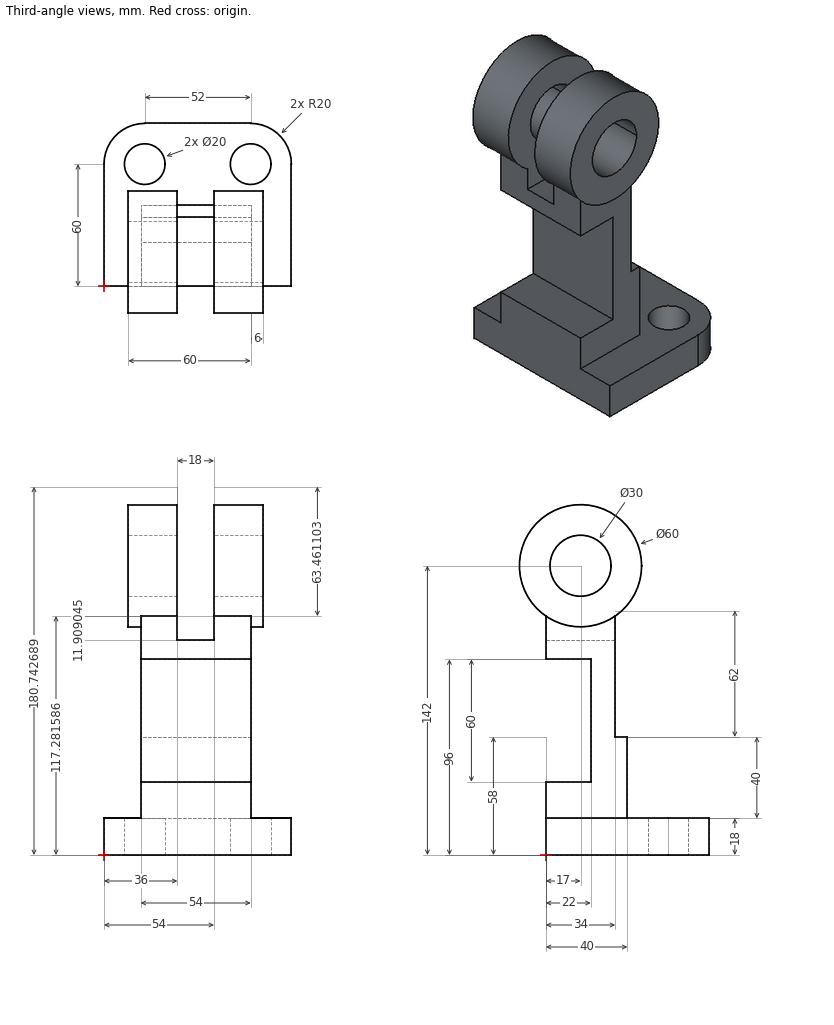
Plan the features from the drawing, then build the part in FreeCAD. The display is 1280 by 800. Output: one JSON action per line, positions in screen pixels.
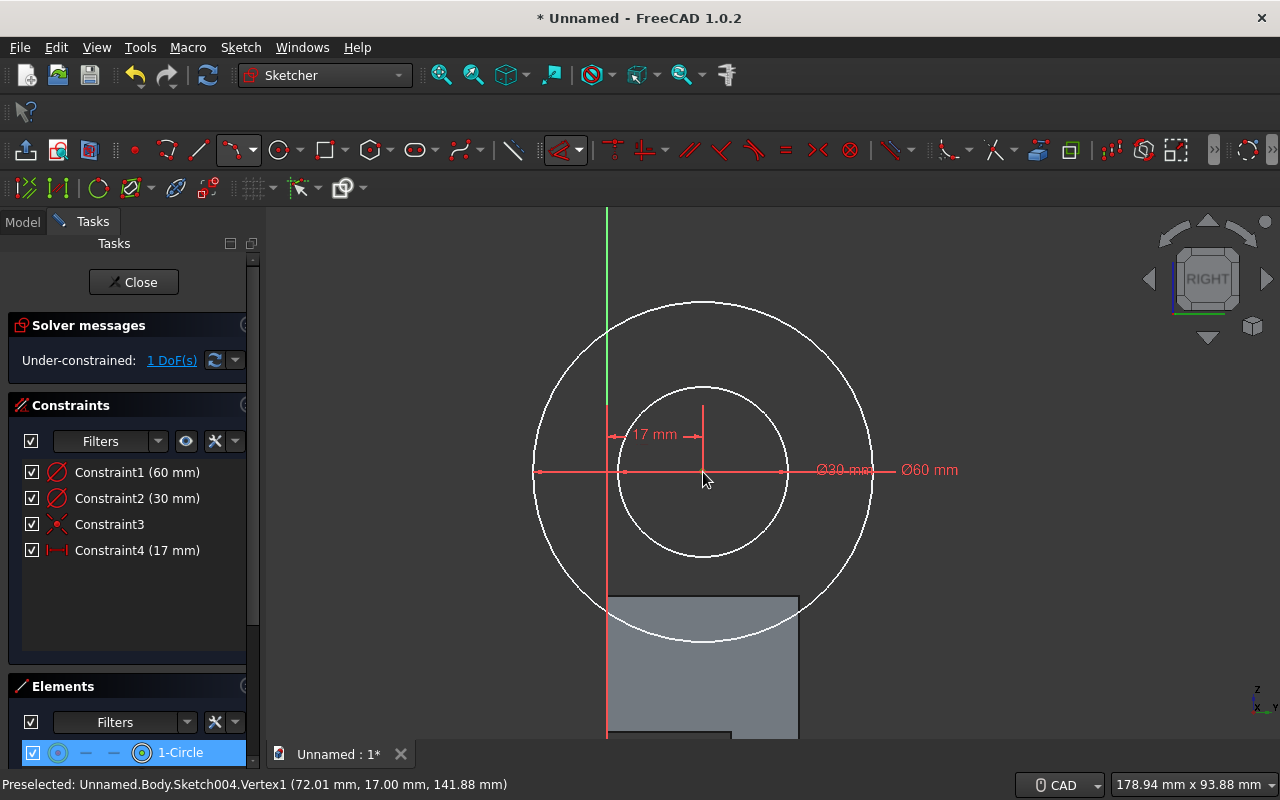
{"action": "left_click", "coordinate": [582, 150]}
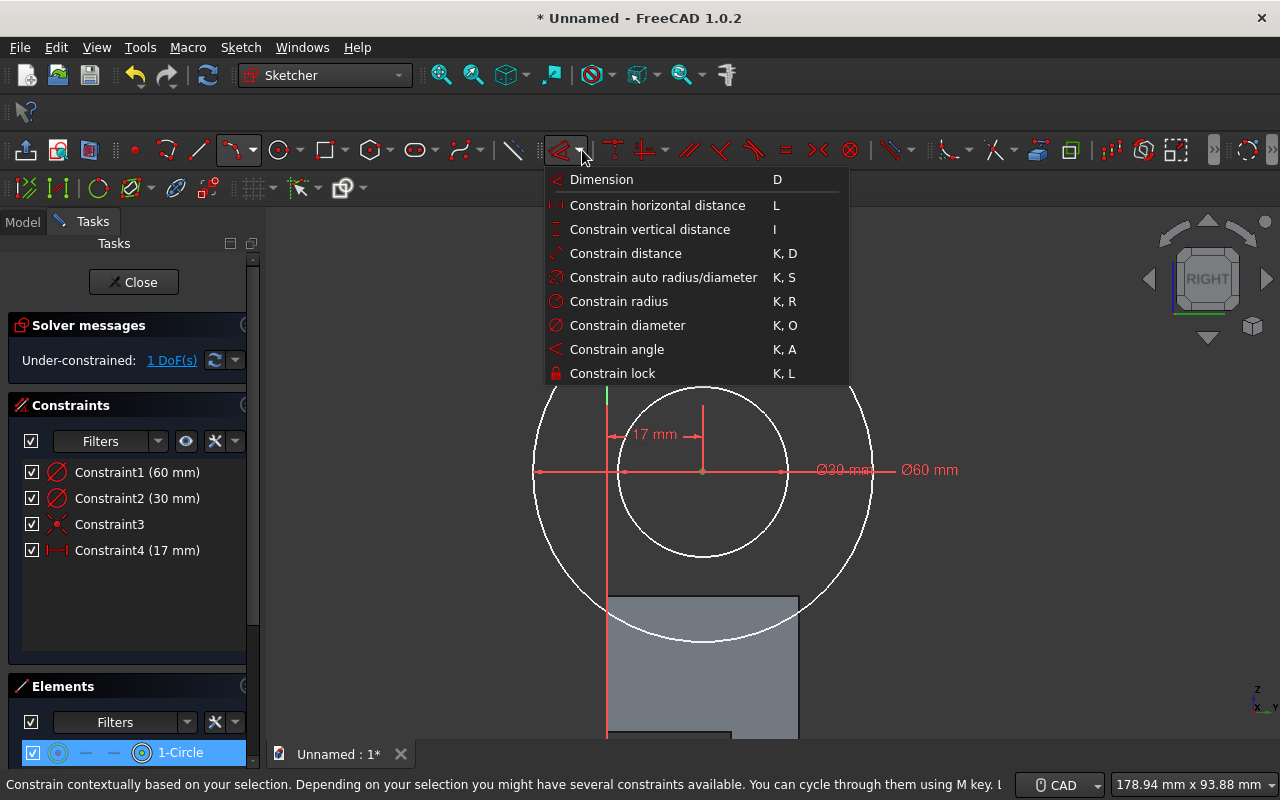
{"action": "left_click", "coordinate": [697, 229]}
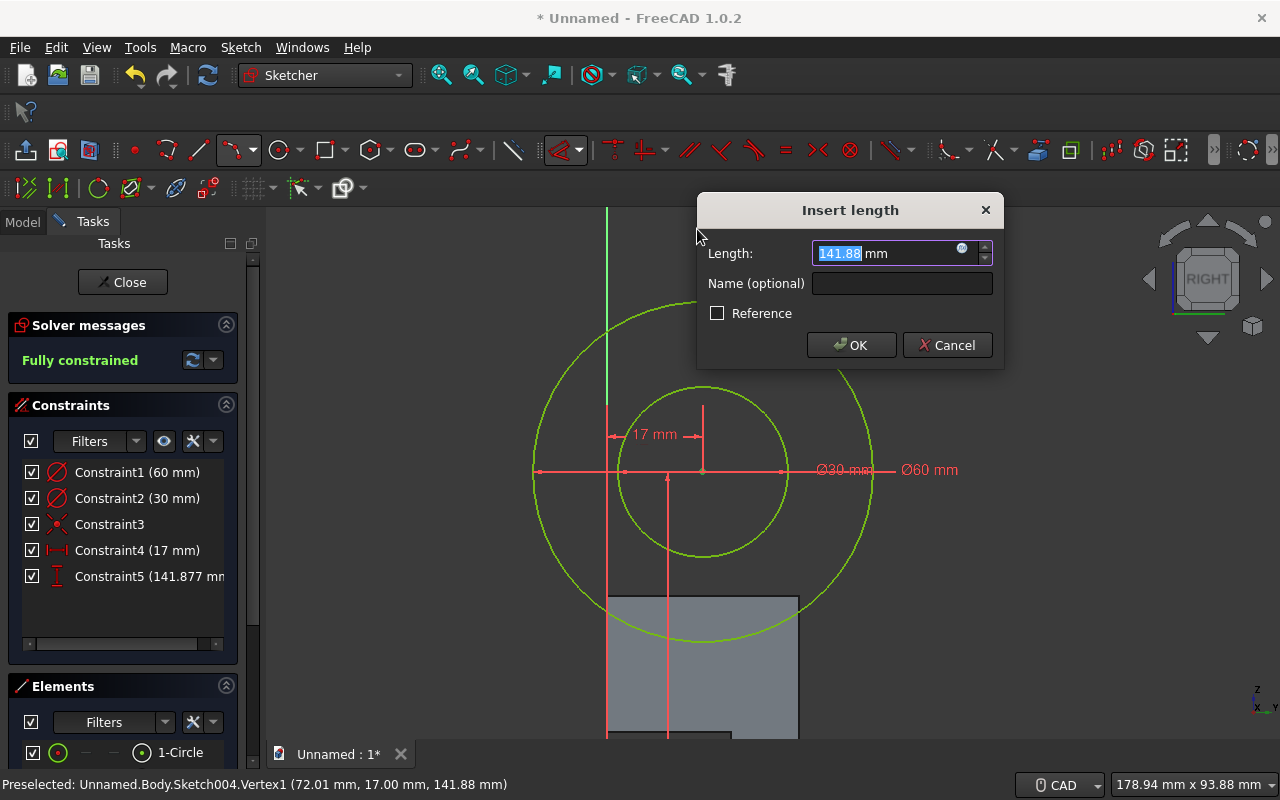
{"action": "type", "text": "142"}
{"action": "key", "text": "Return"}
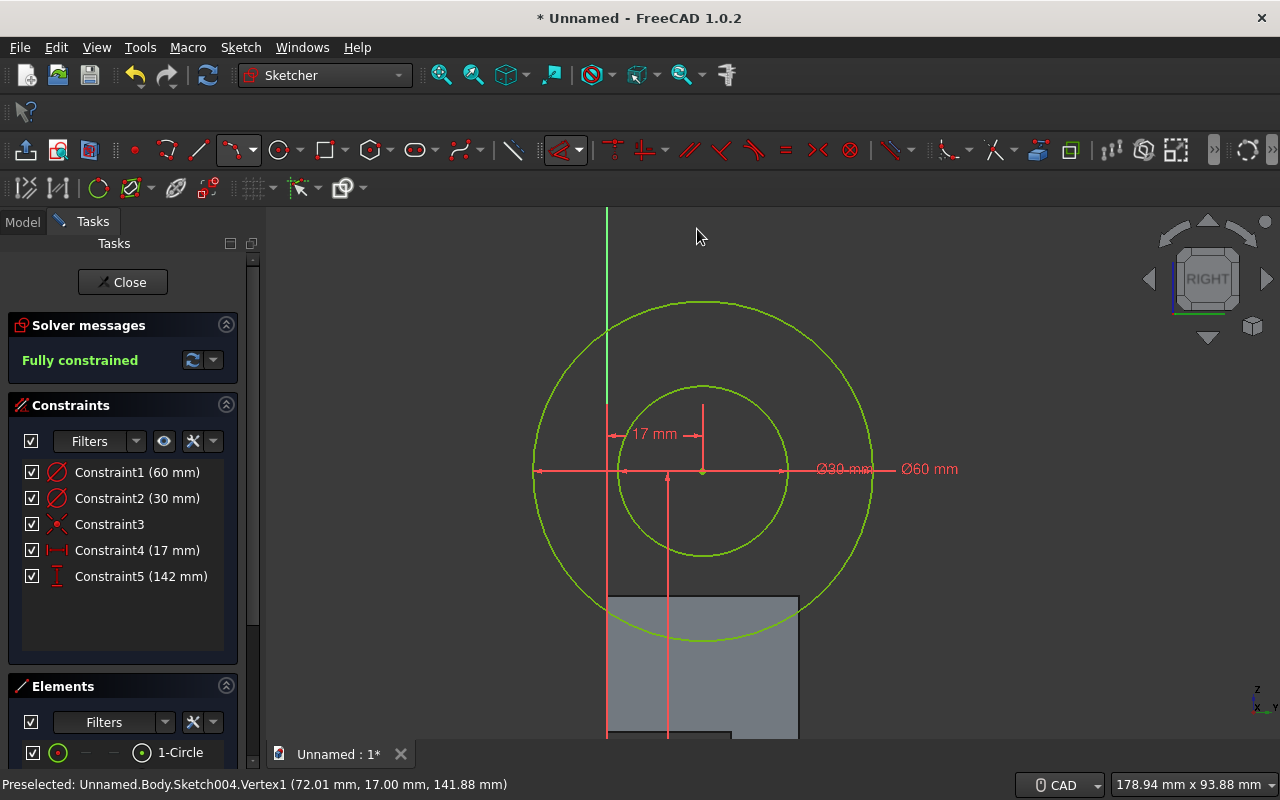
{"action": "left_click", "coordinate": [123, 282]}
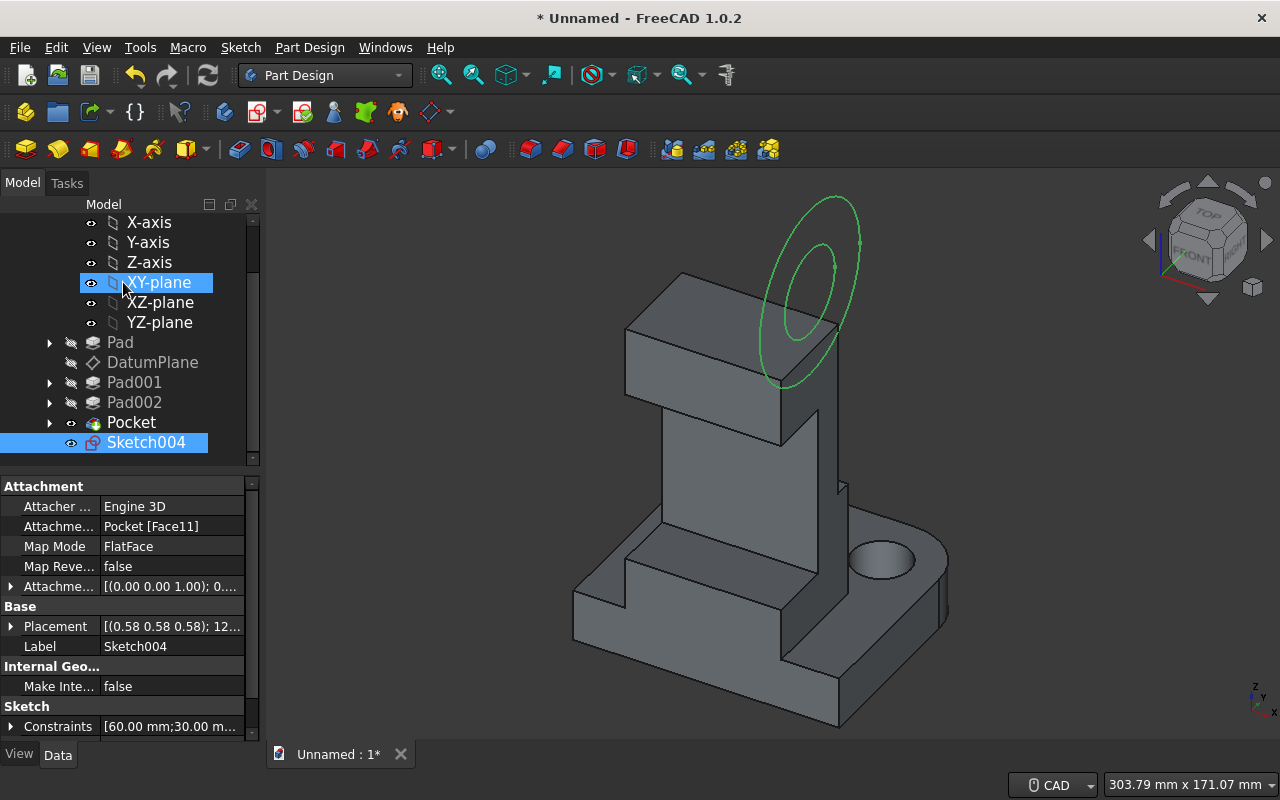
{"action": "left_click", "coordinate": [26, 150]}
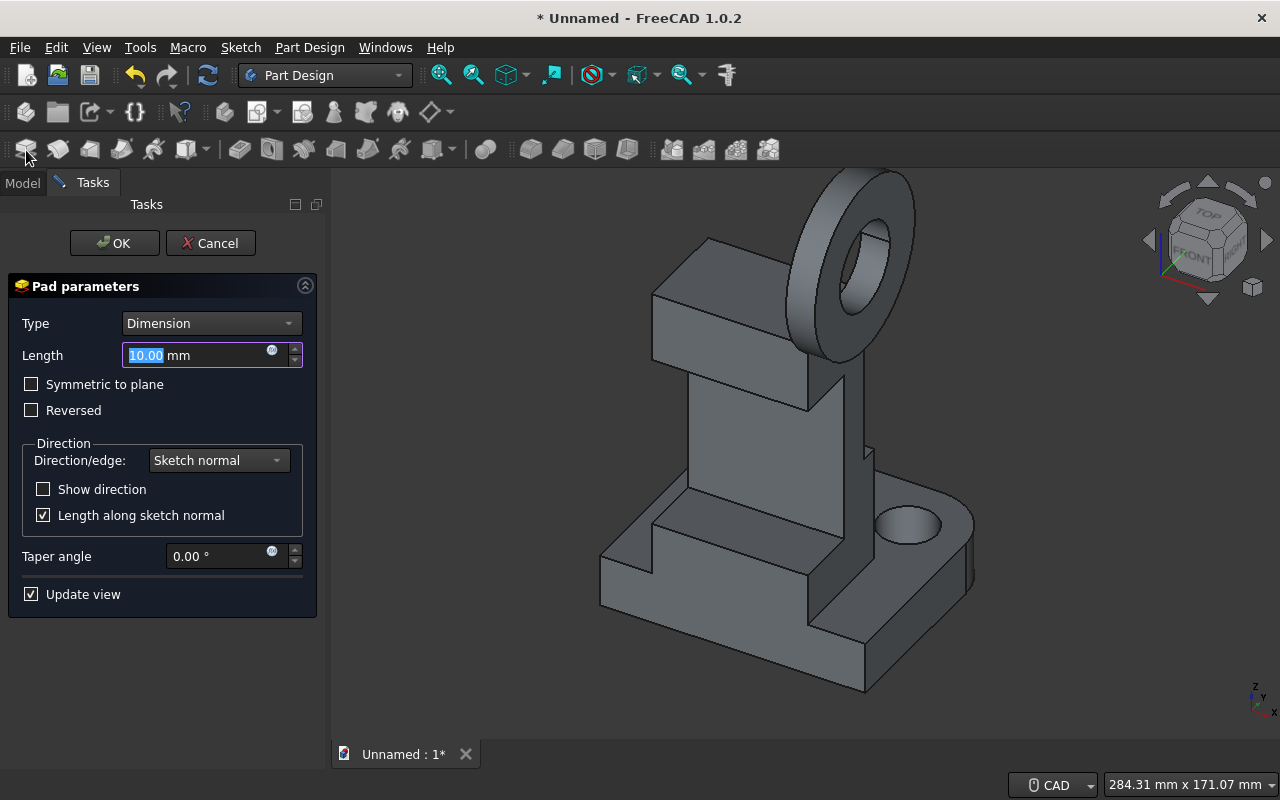
{"action": "left_click", "coordinate": [212, 324]}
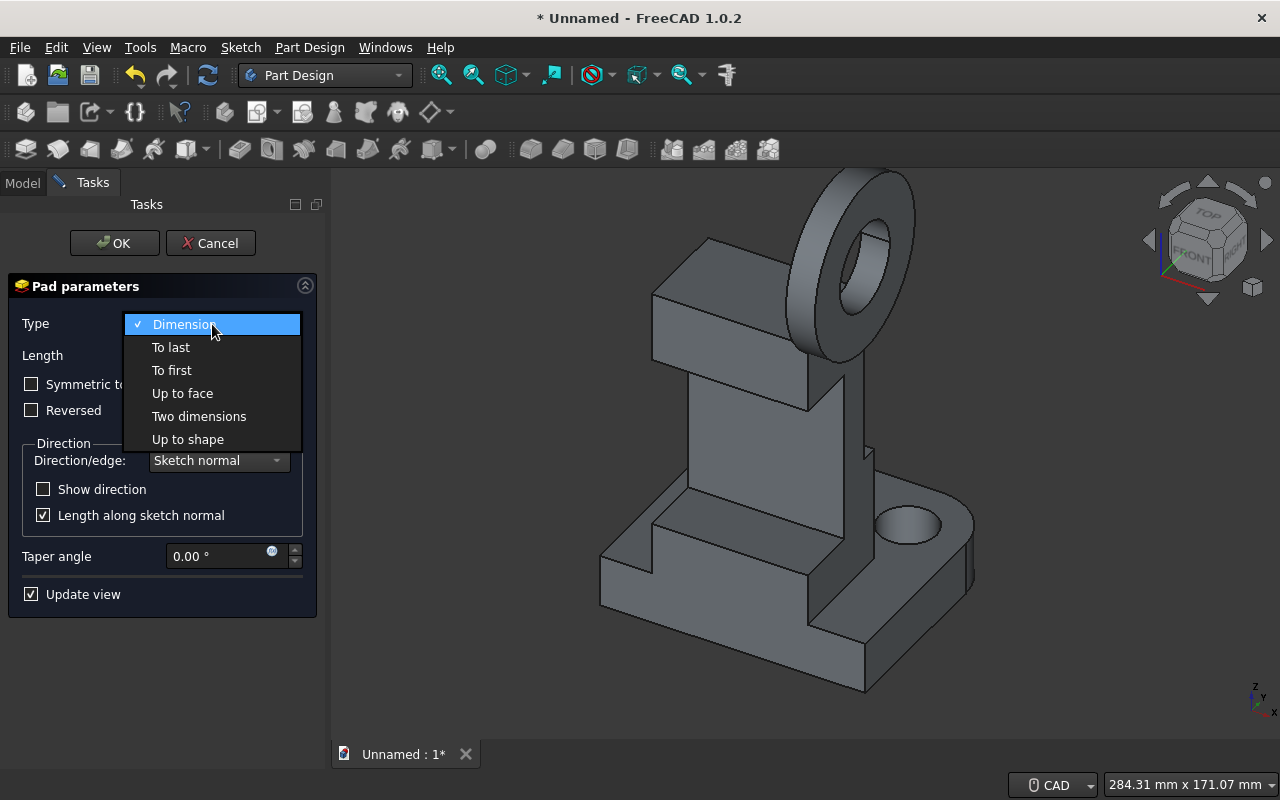
{"action": "left_click", "coordinate": [212, 416]}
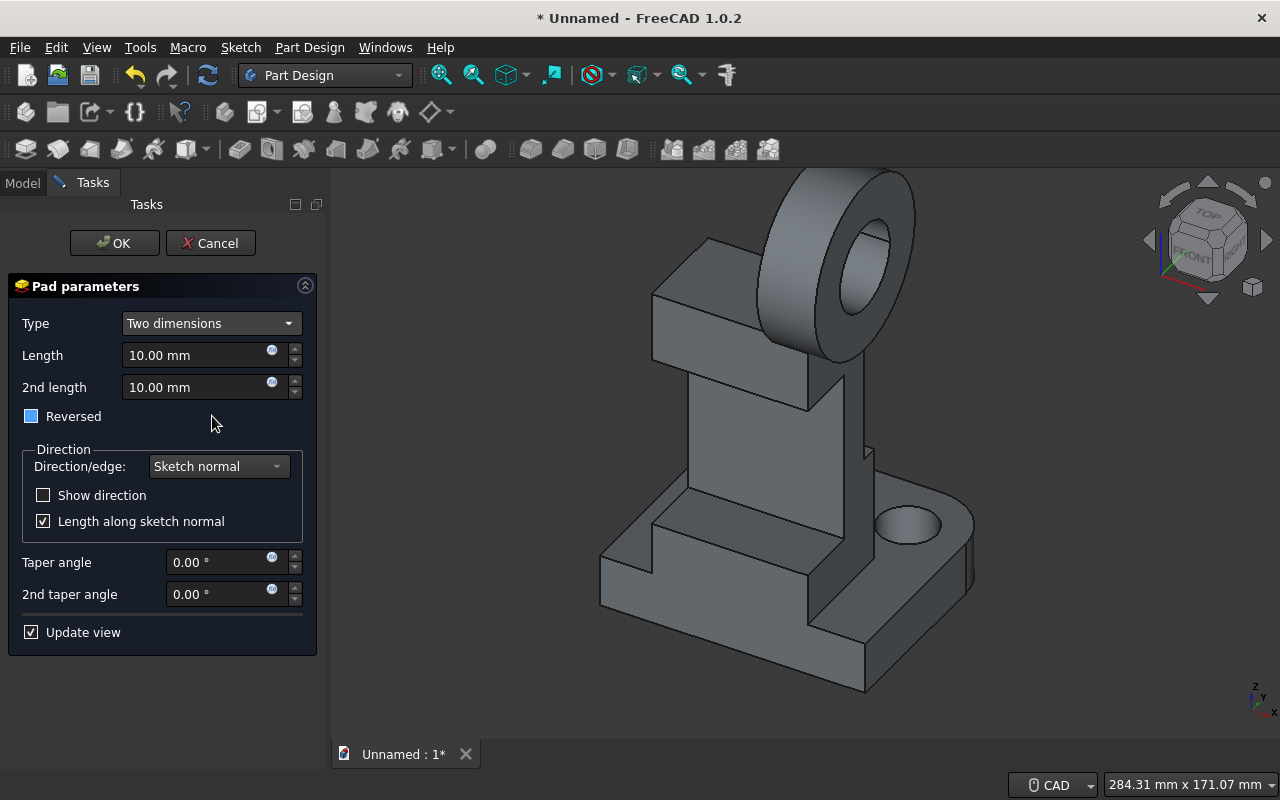
{"action": "triple_click", "coordinate": [204, 355]}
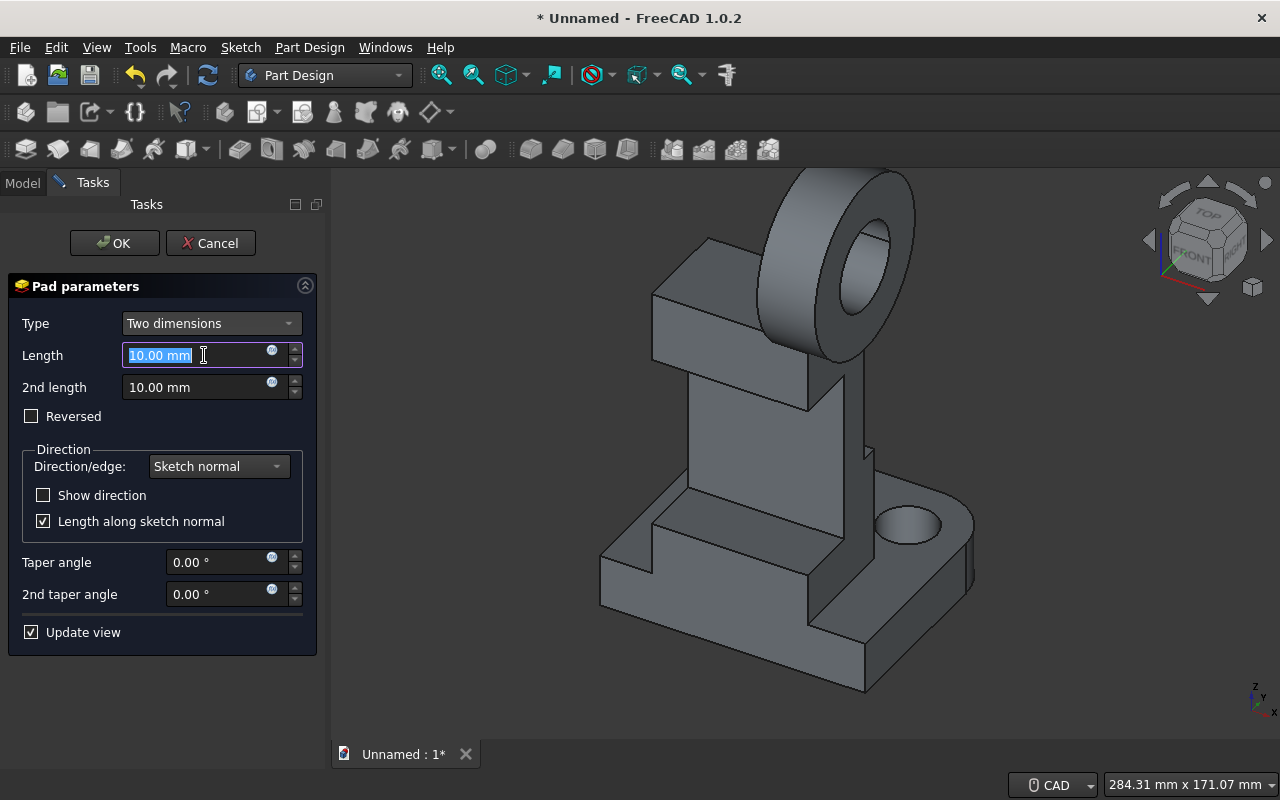
{"action": "type", "text": "6"}
{"action": "key", "text": "Tab"}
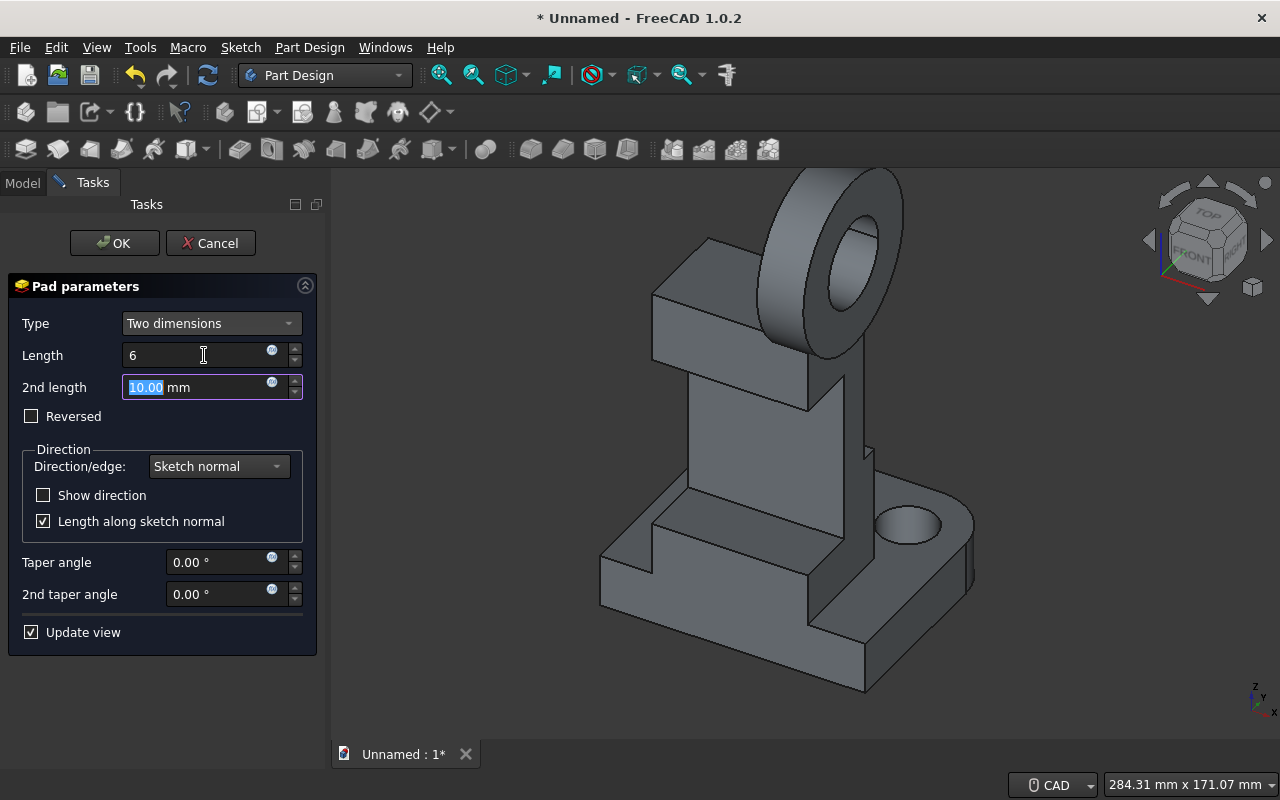
{"action": "type", "text": "60"}
{"action": "key", "text": "Tab"}